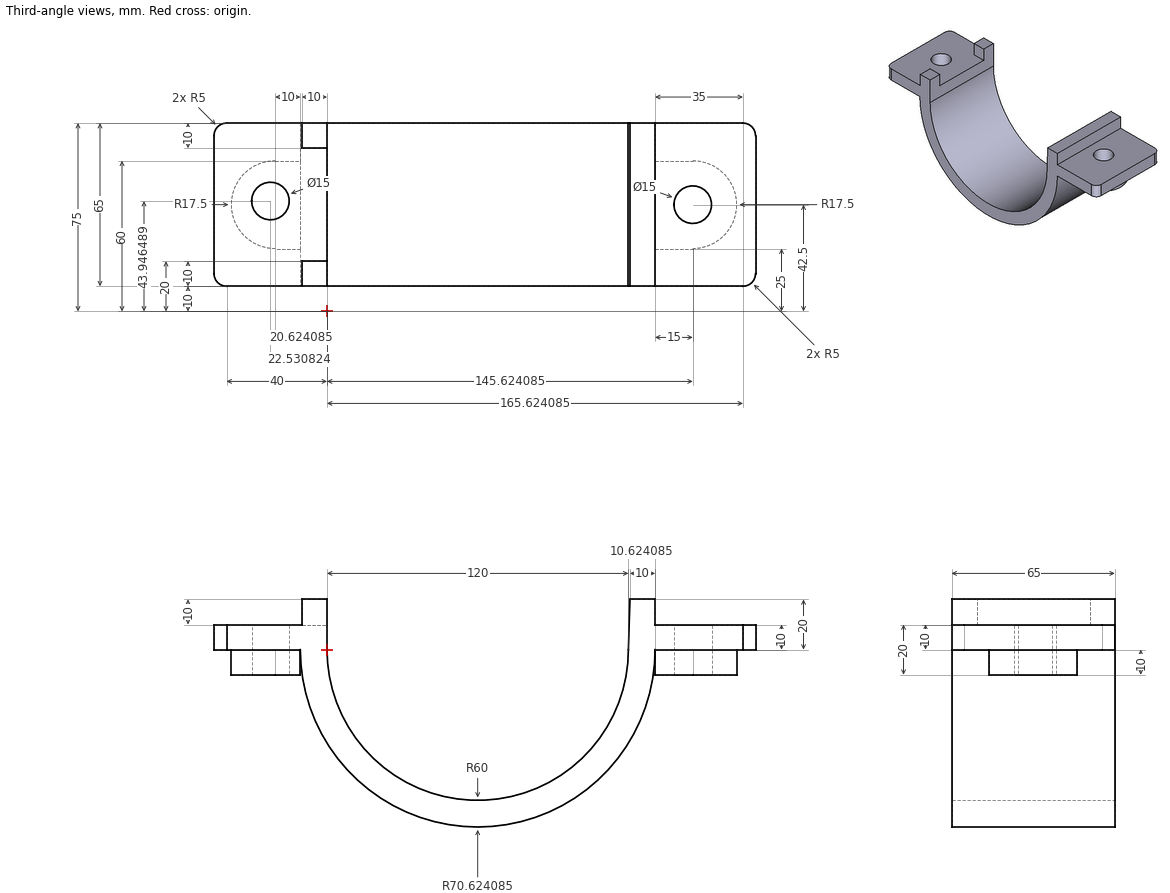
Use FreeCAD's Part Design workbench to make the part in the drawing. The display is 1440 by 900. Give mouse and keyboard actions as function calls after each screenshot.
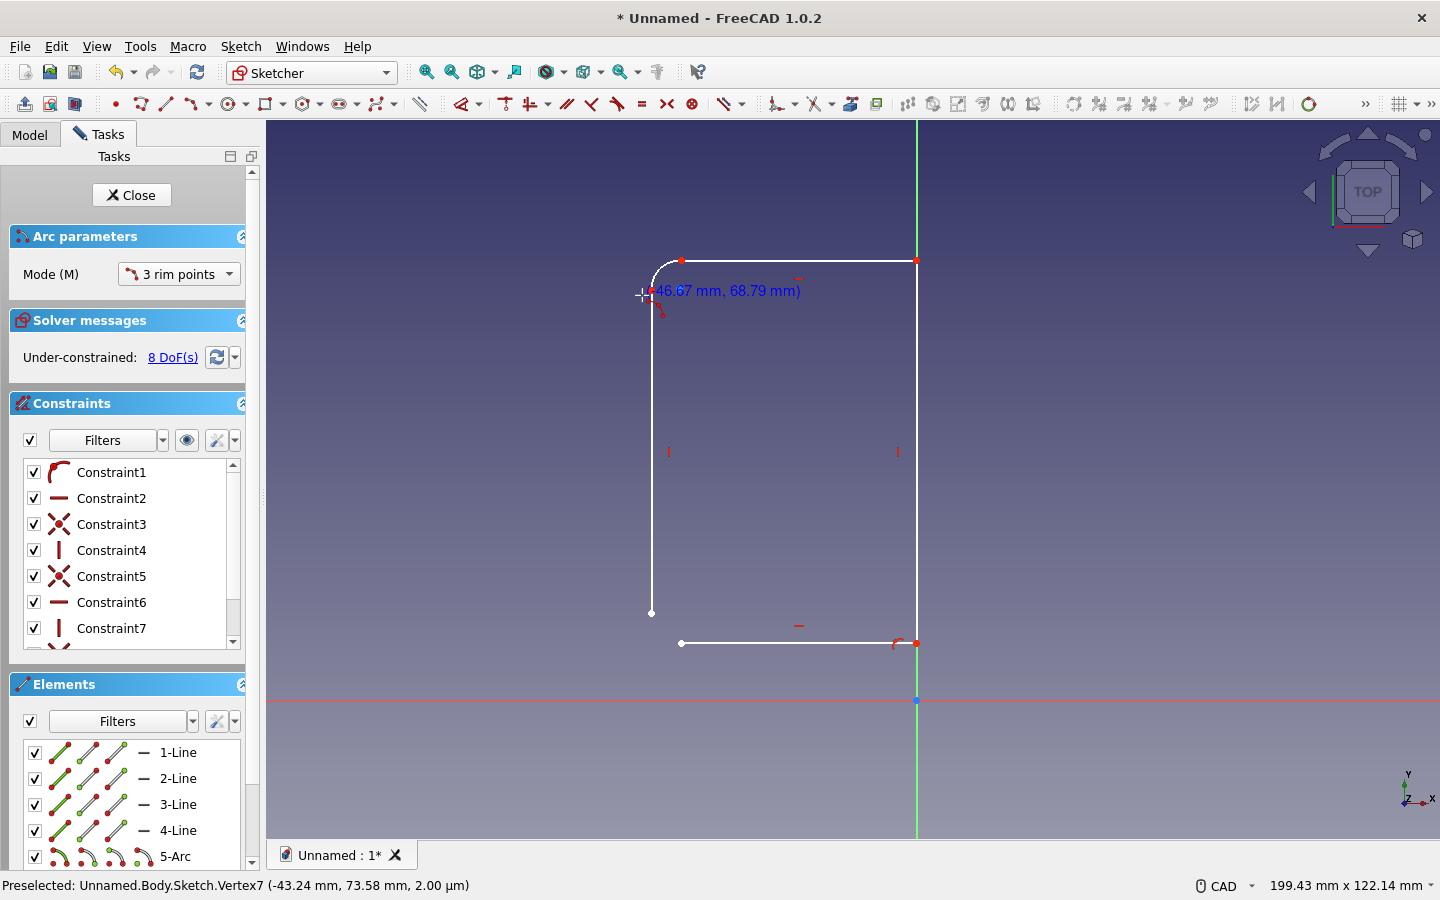
click(652, 614)
click(681, 643)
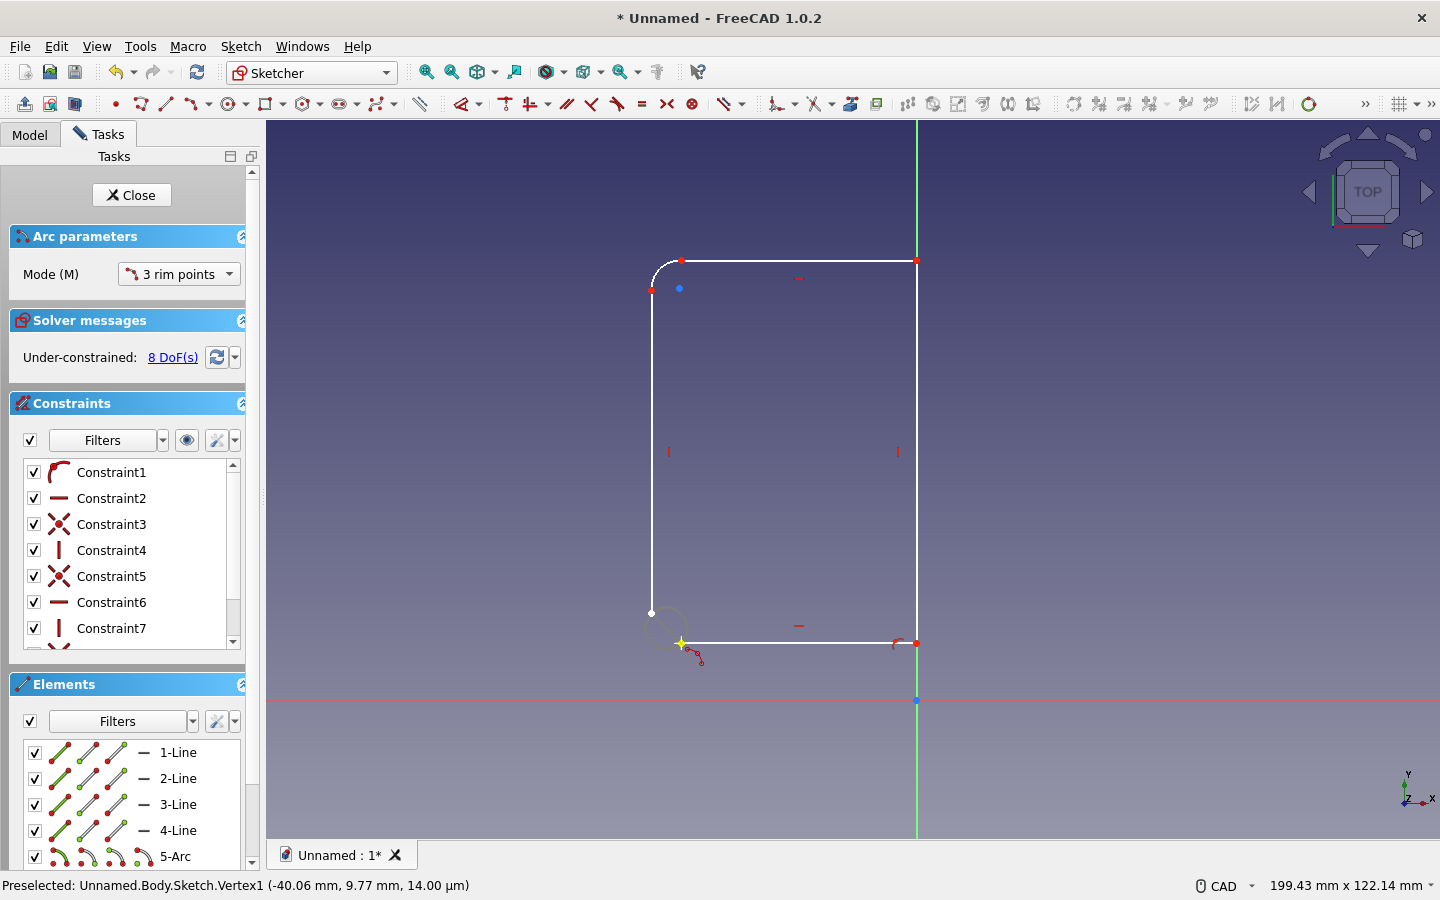
scroll(661, 633, up, 4)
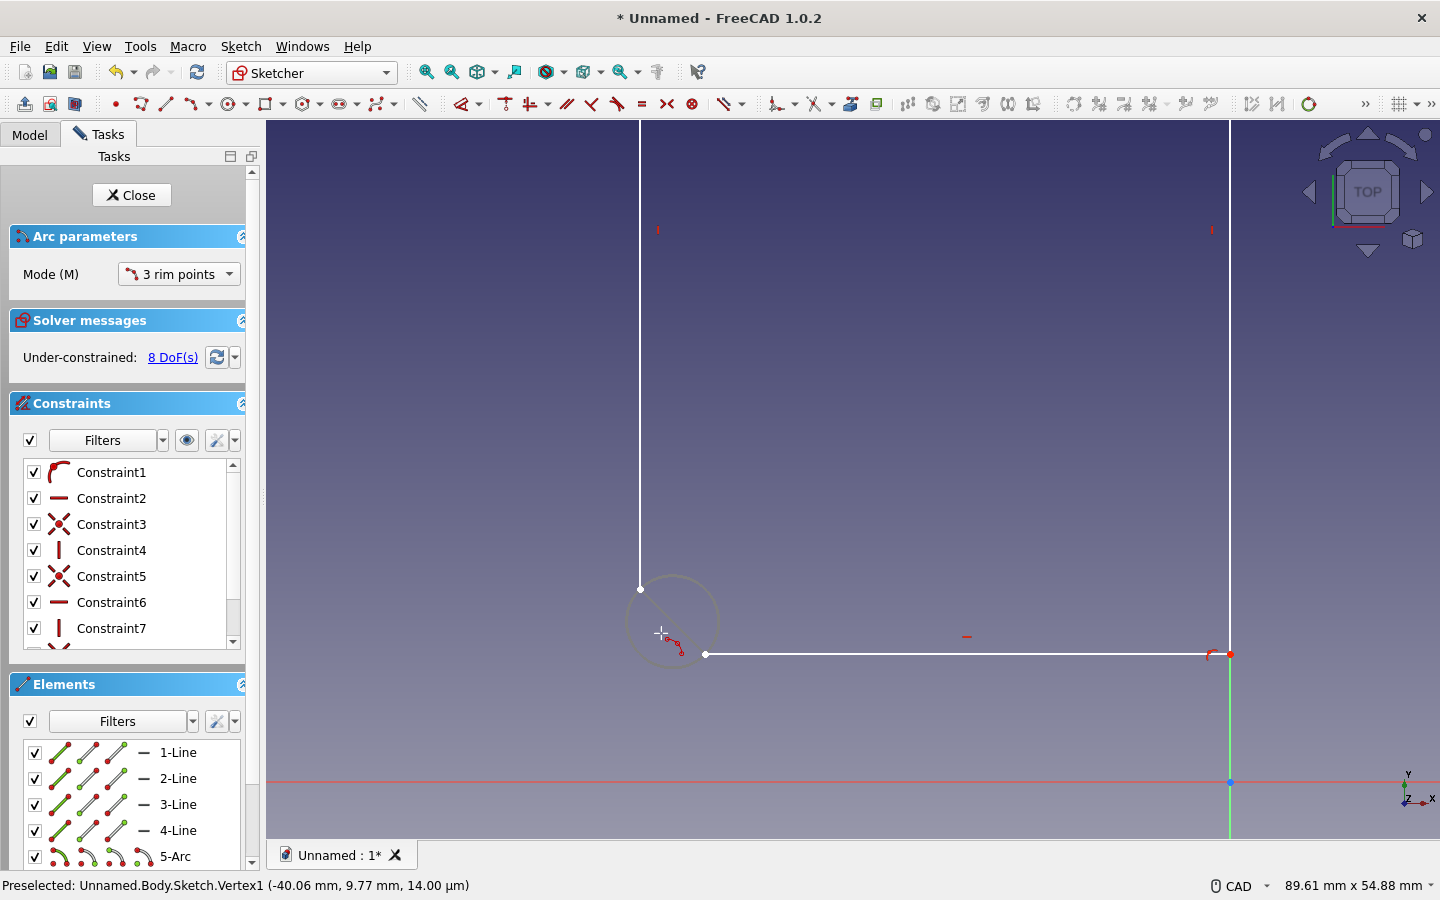
click(660, 632)
key(Escape)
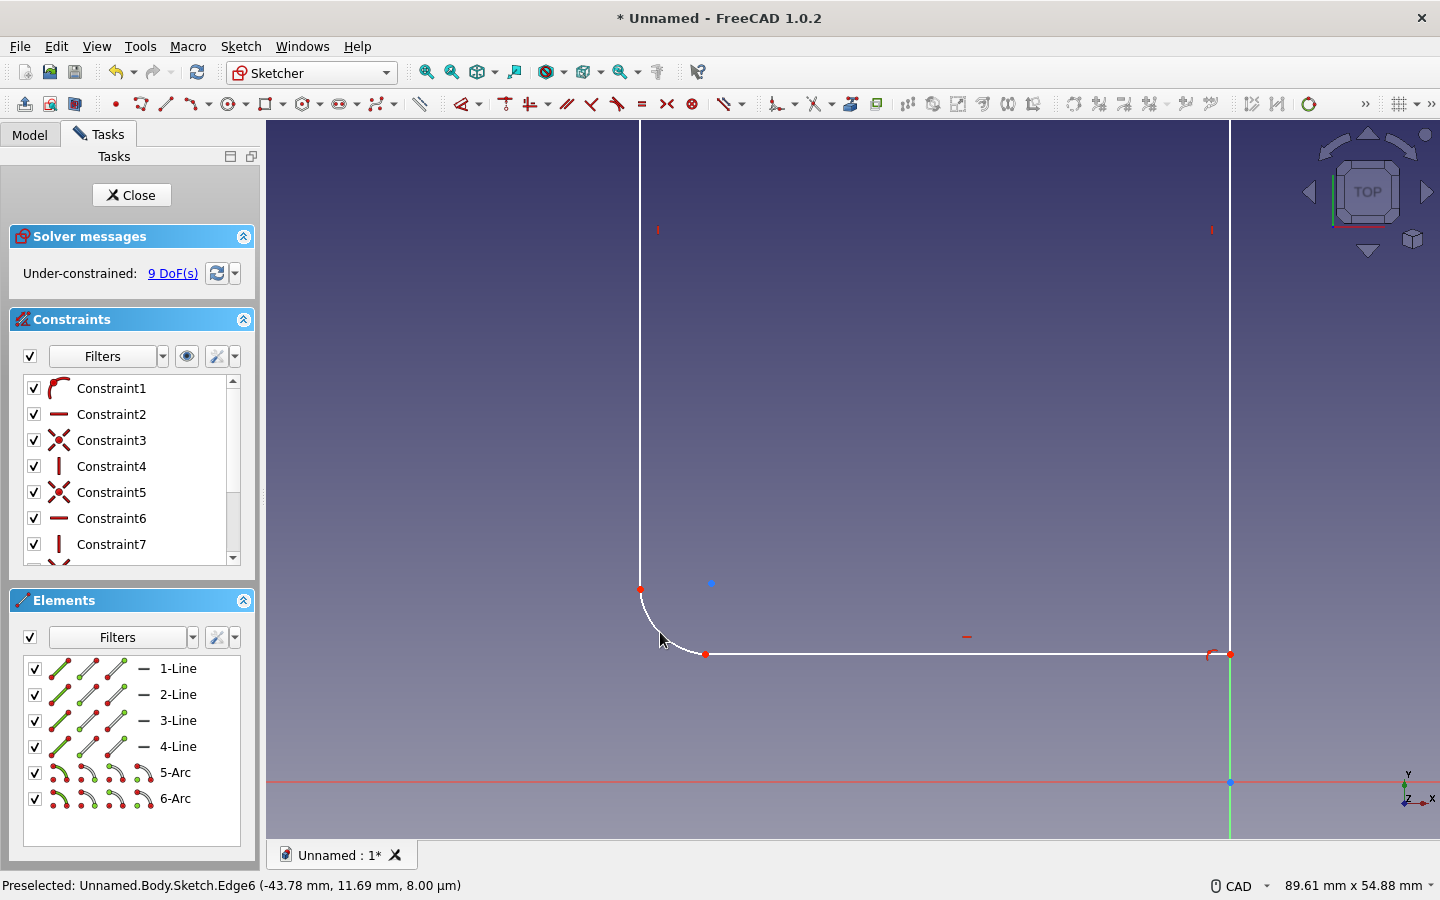
click(863, 654)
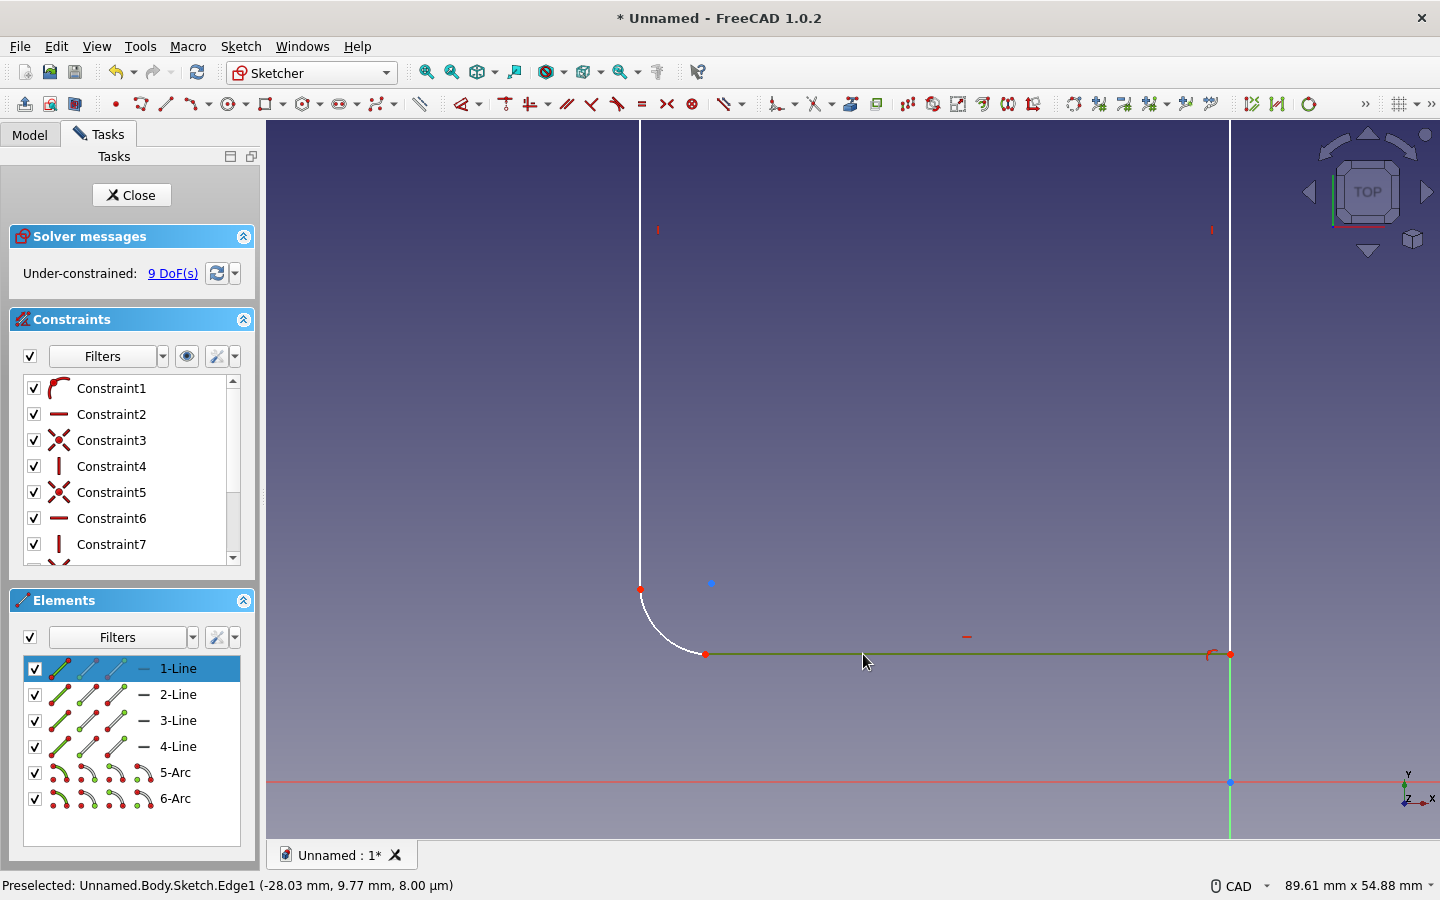
click(649, 618)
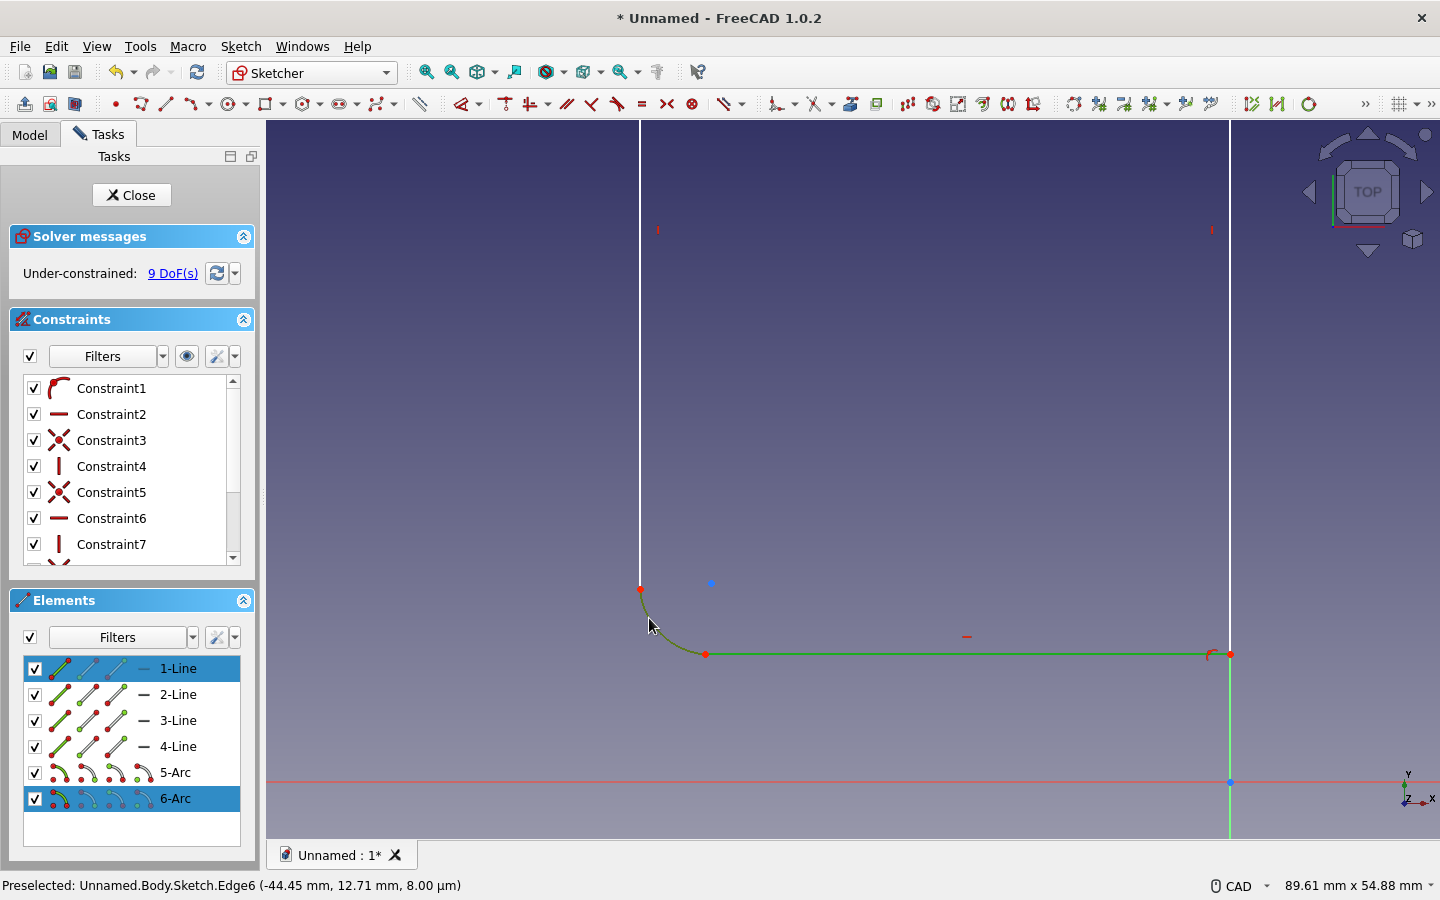
key(t)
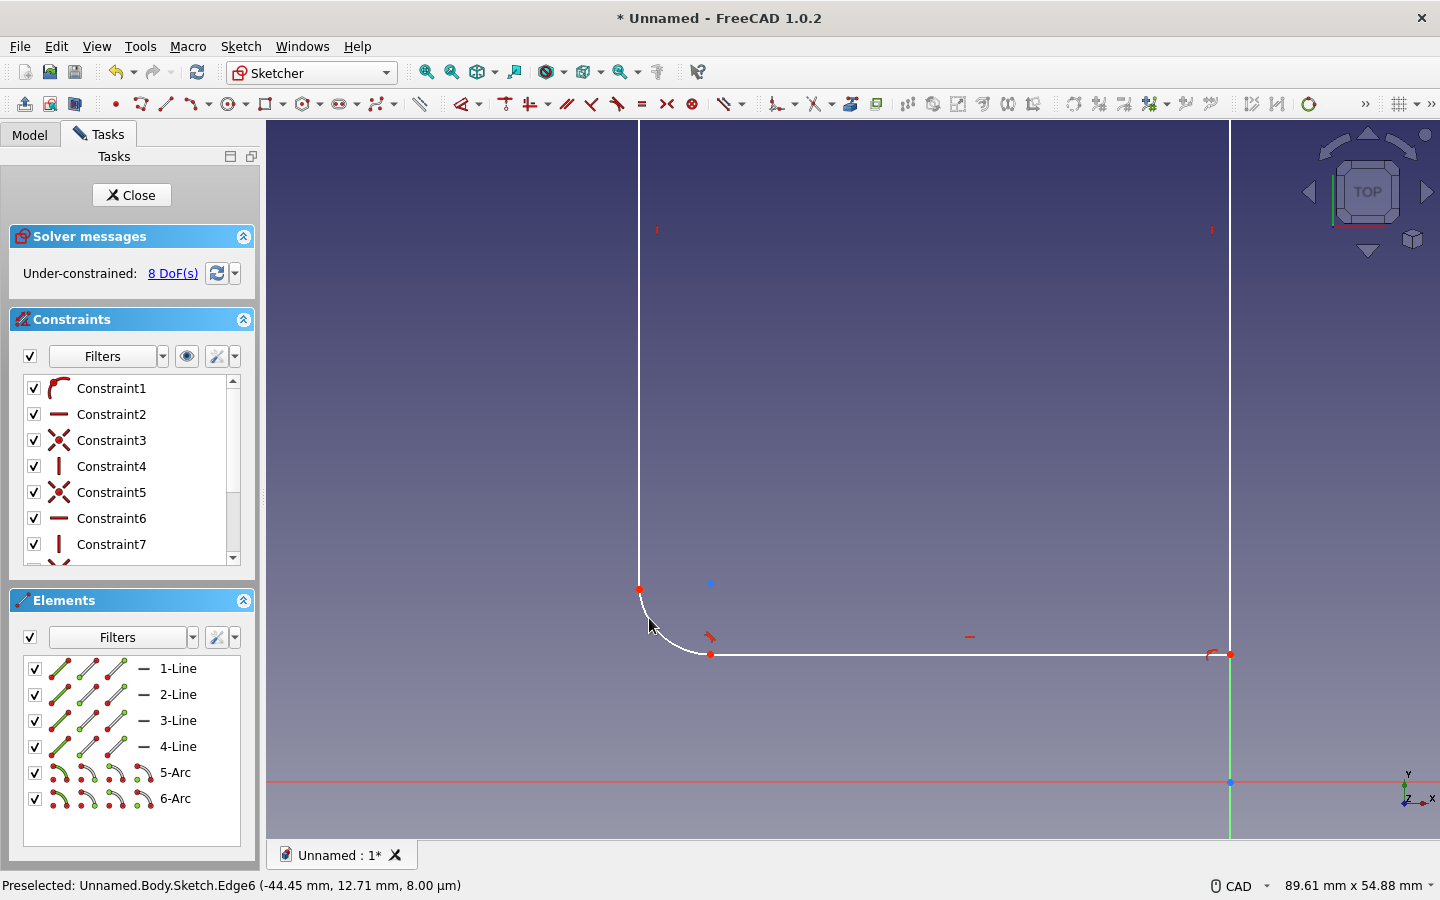
scroll(661, 633, down, 4)